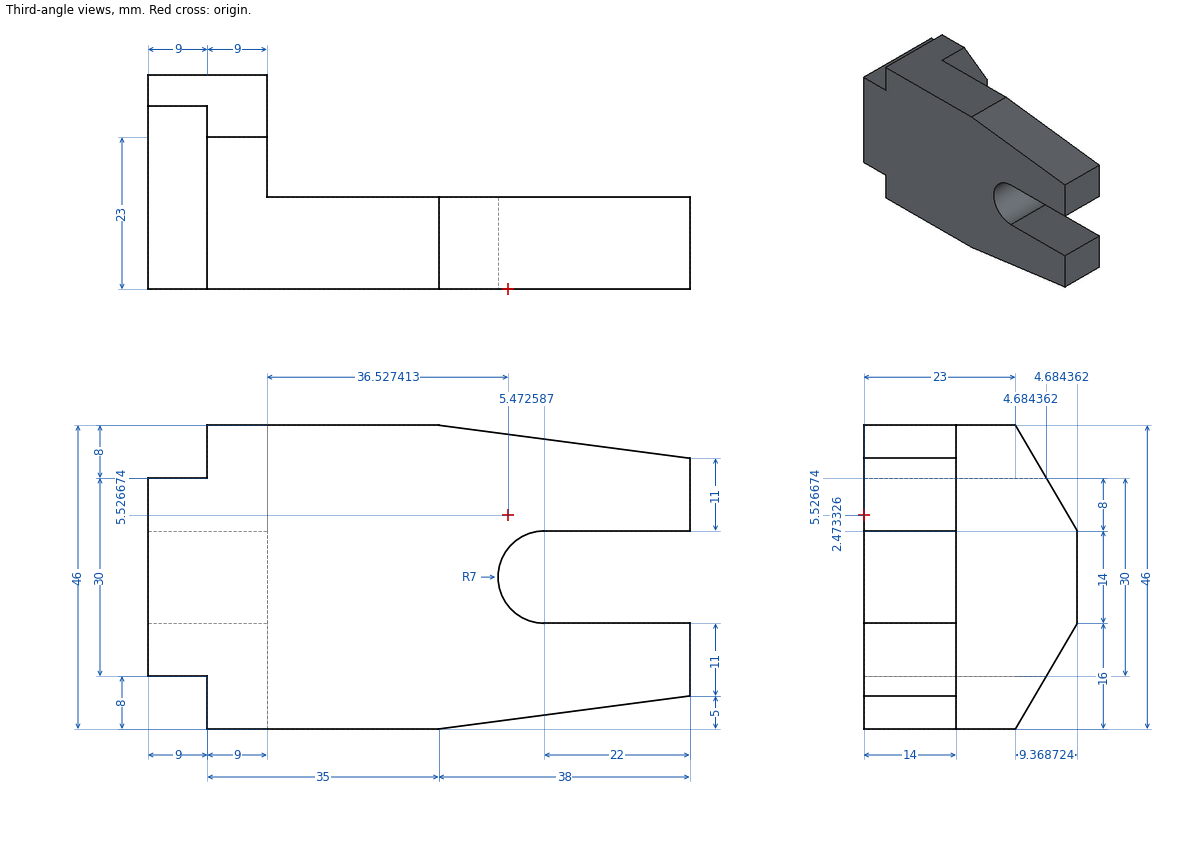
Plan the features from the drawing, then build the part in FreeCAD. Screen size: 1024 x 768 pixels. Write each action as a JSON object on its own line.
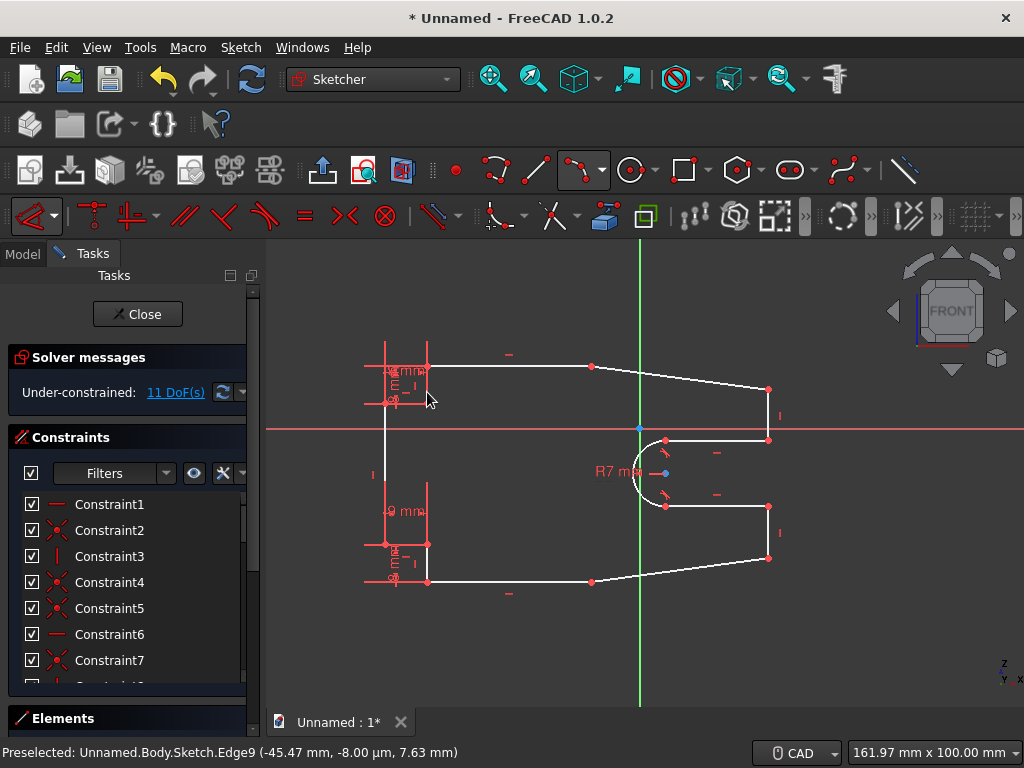
{"action": "left_click", "coordinate": [697, 506]}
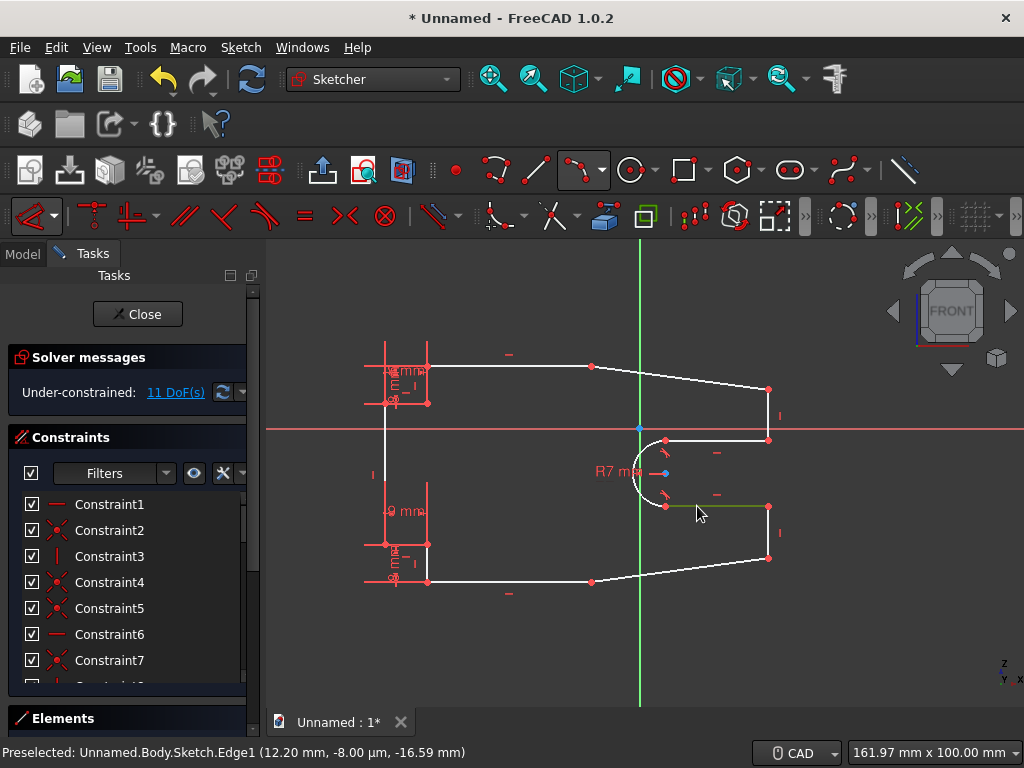
{"action": "key", "text": "l"}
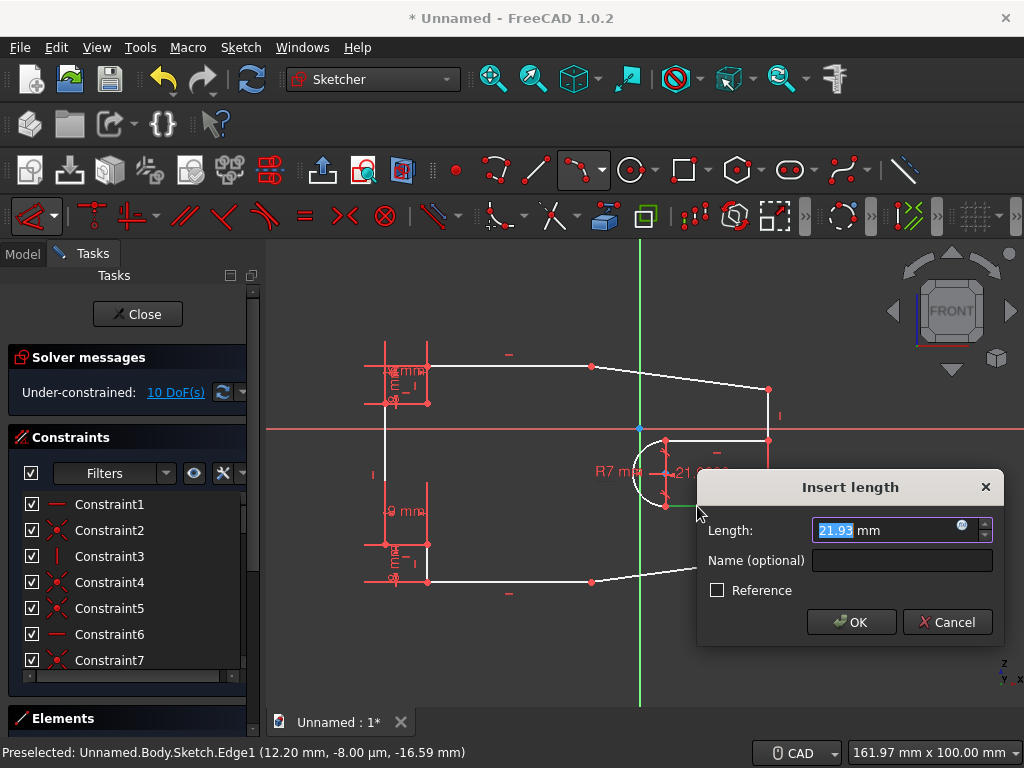
{"action": "type", "text": "22"}
{"action": "key", "text": "Return"}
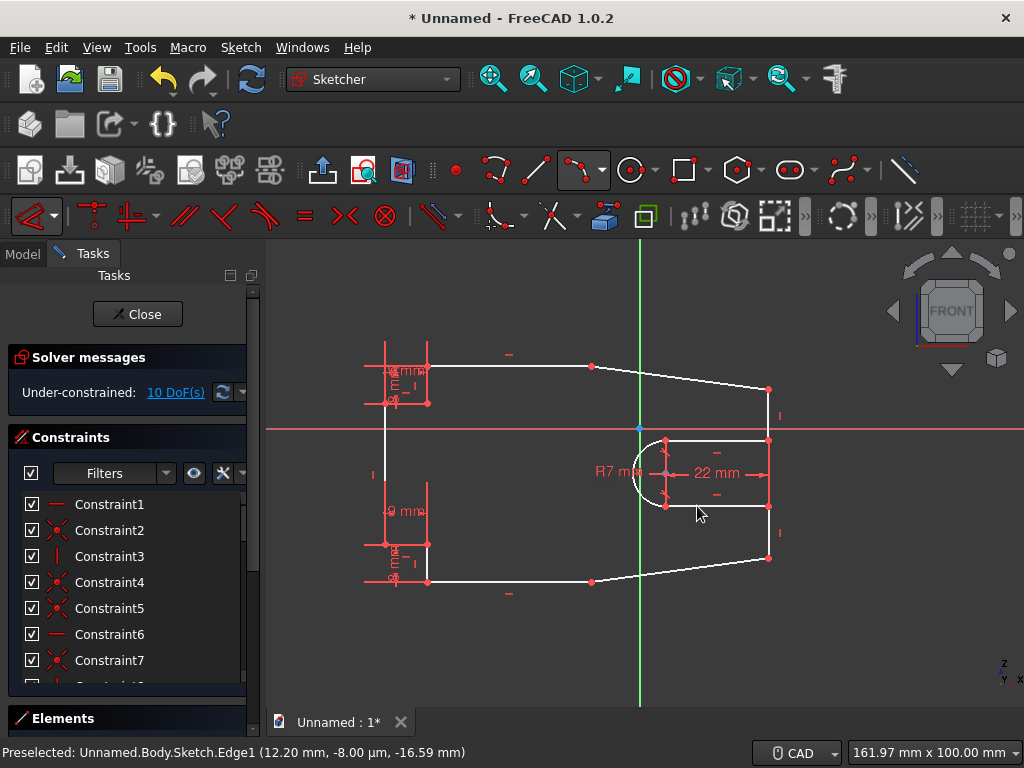
{"action": "left_click", "coordinate": [769, 522]}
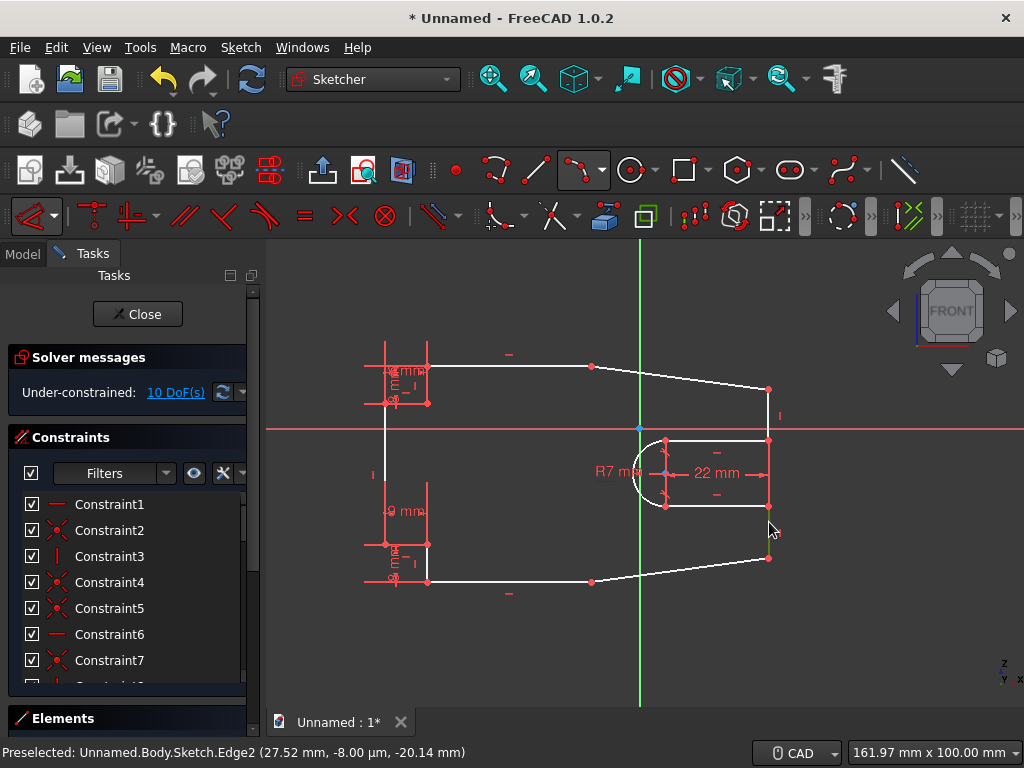
{"action": "left_click", "coordinate": [56, 216]}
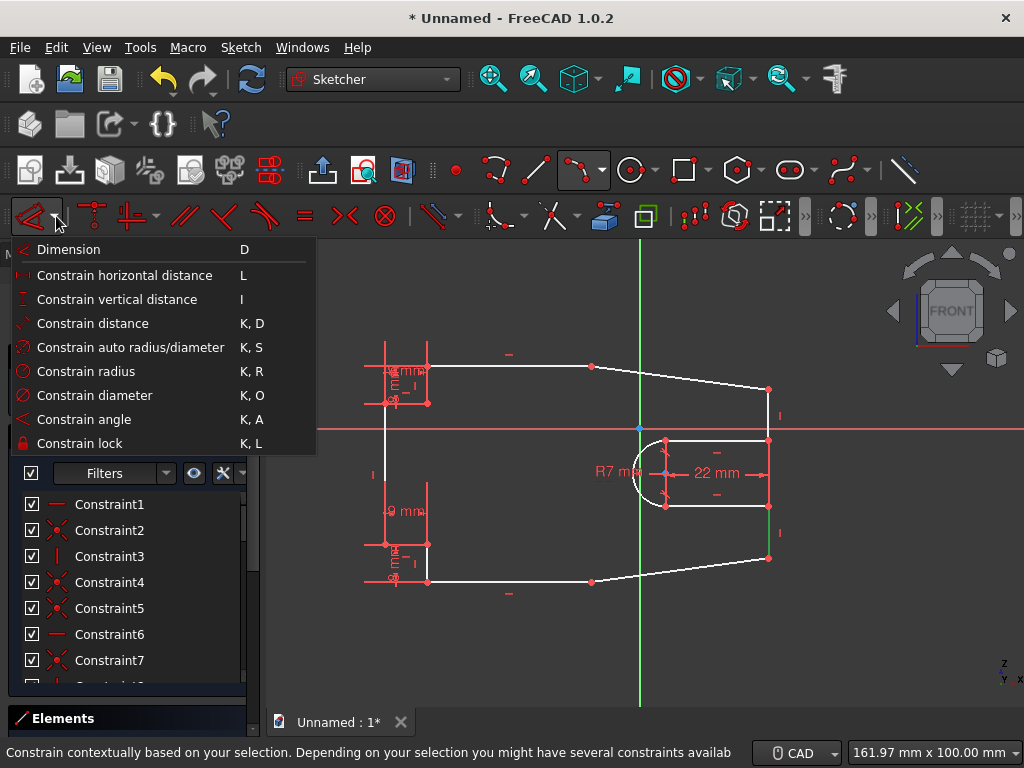
{"action": "left_click", "coordinate": [164, 299]}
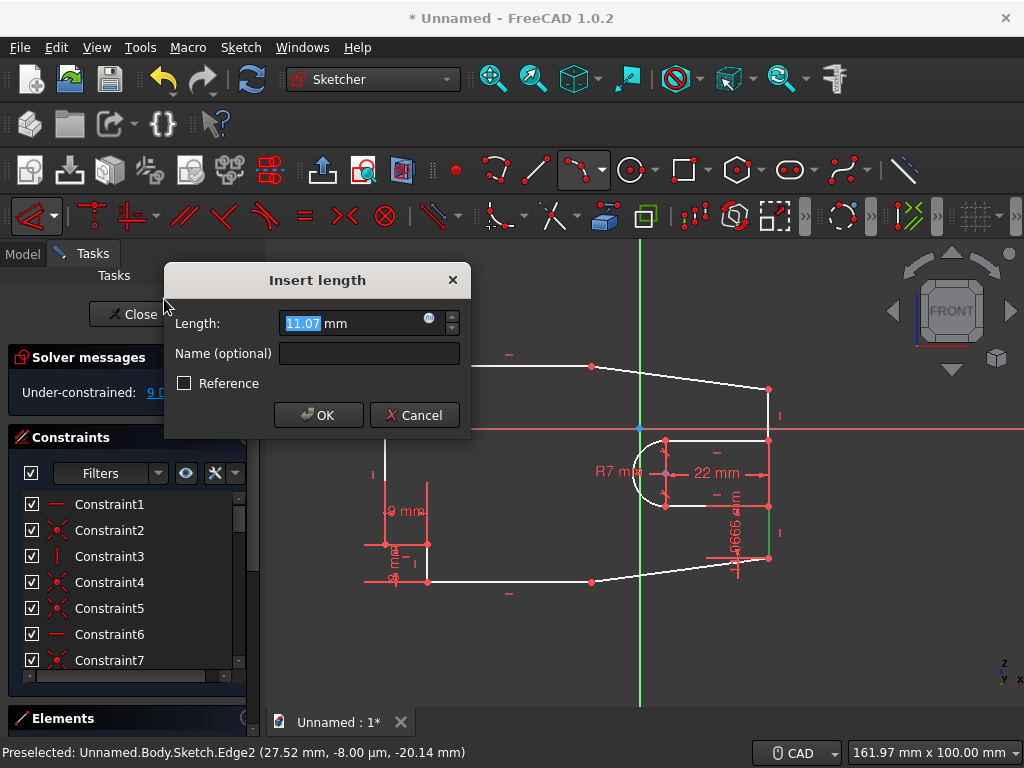
{"action": "type", "text": "11"}
{"action": "key", "text": "Return"}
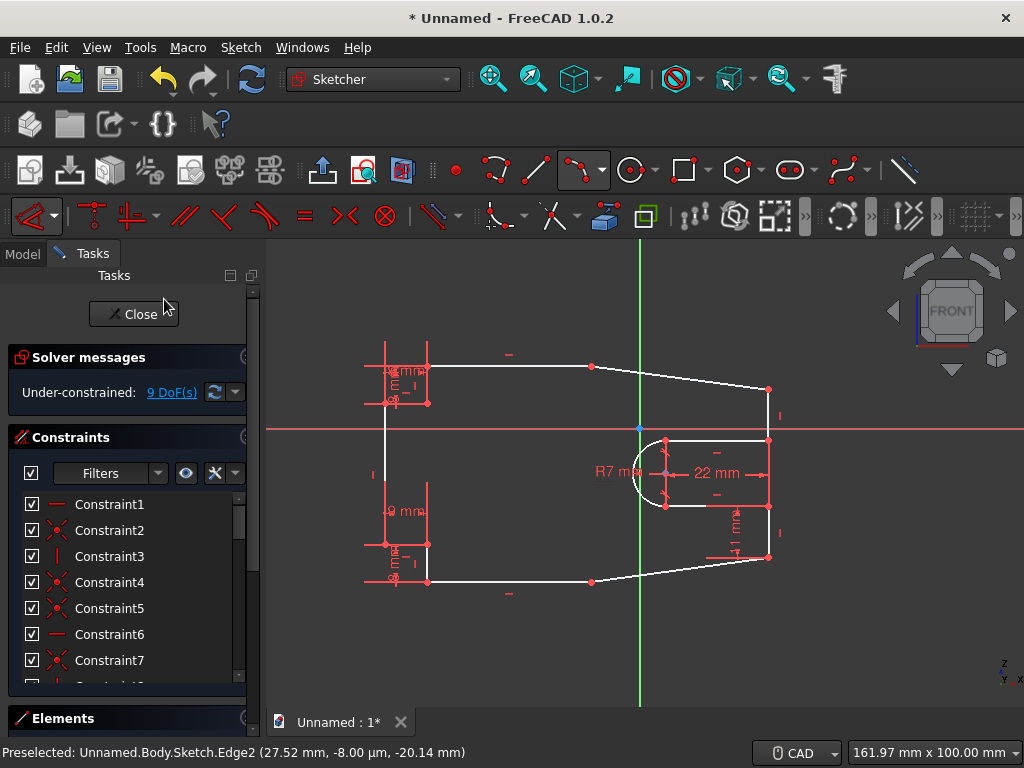
{"action": "left_click", "coordinate": [542, 582]}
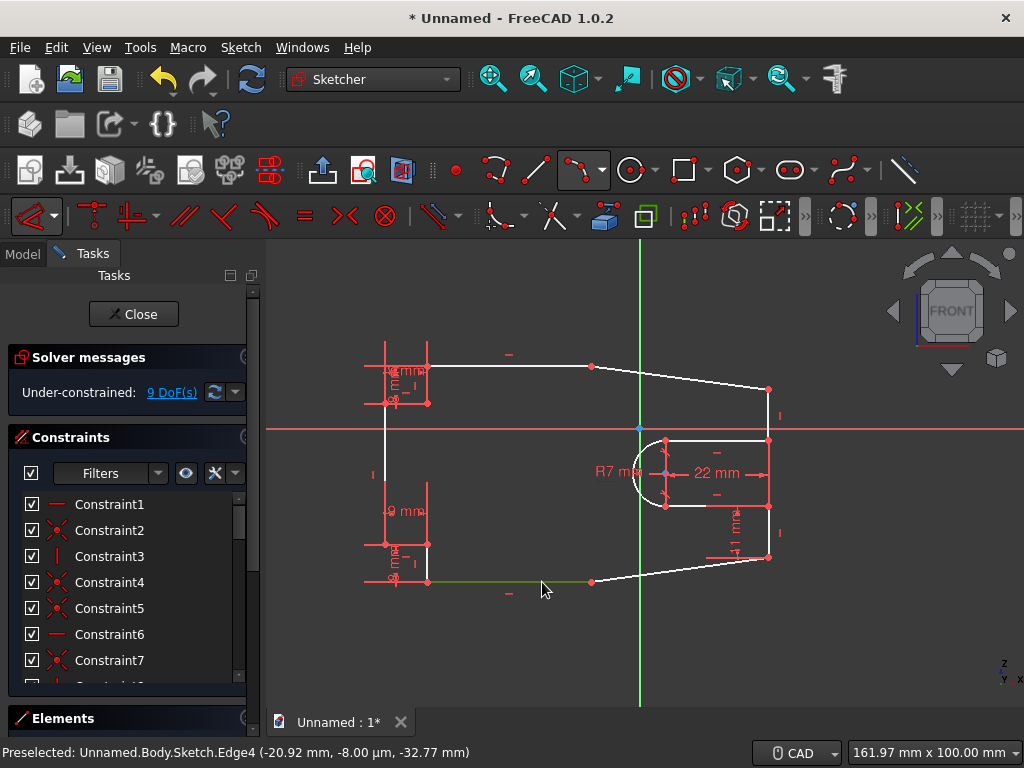
{"action": "left_click", "coordinate": [56, 216]}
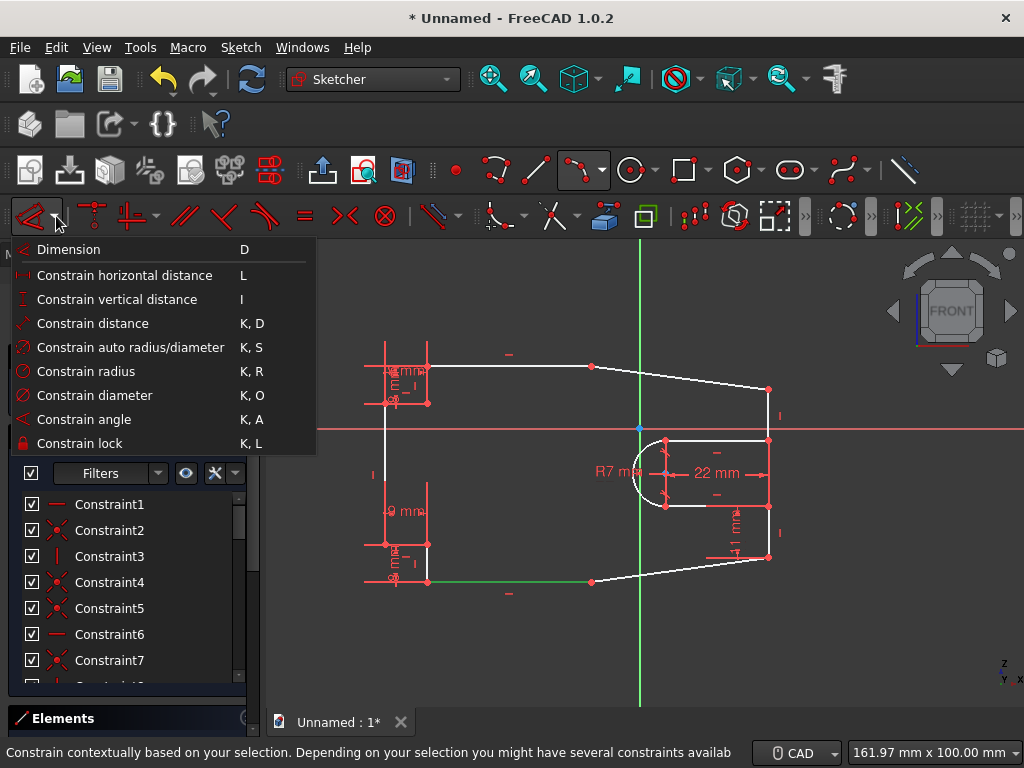
{"action": "left_click", "coordinate": [164, 275]}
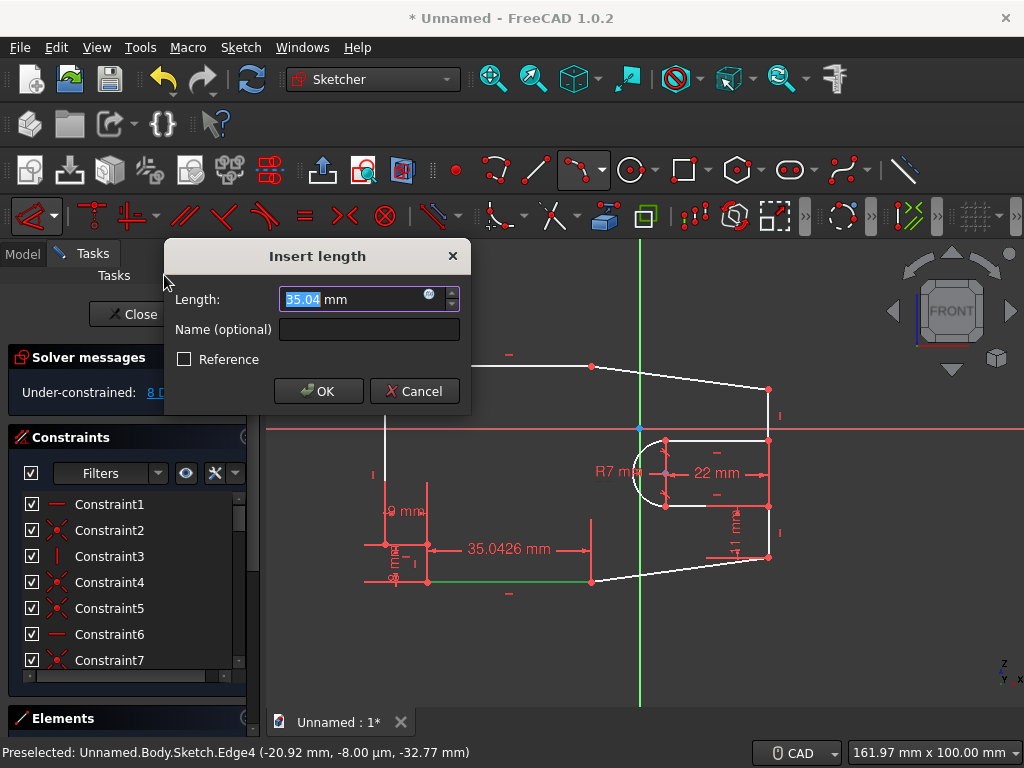
{"action": "type", "text": "35"}
{"action": "key", "text": "Return"}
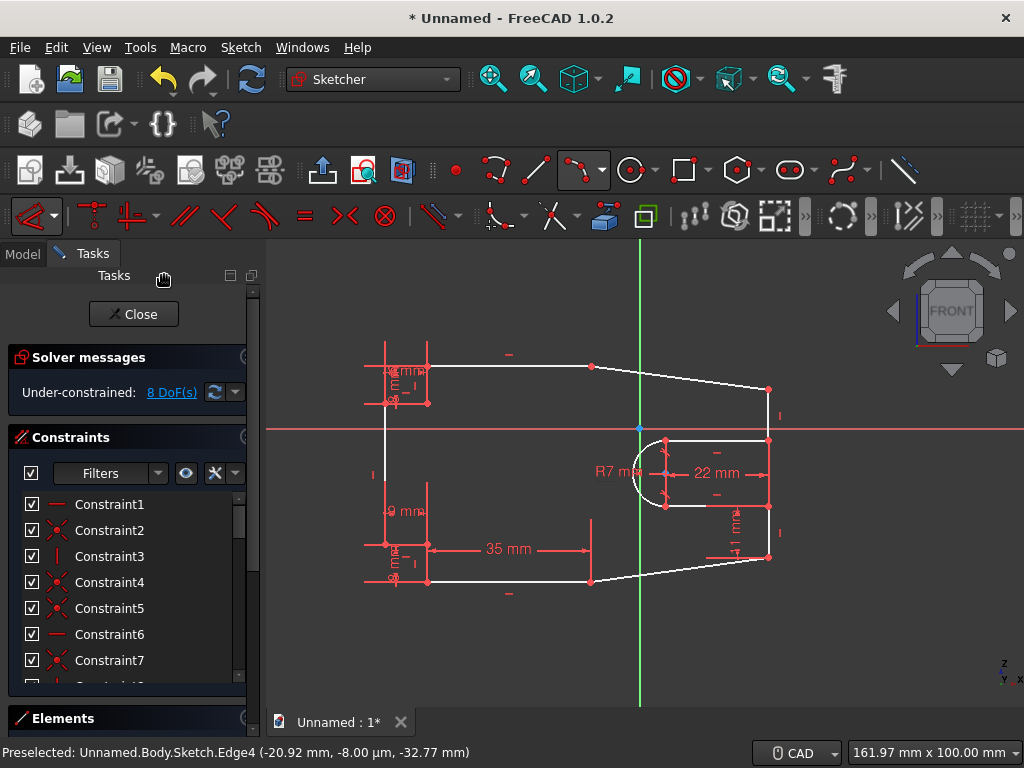
{"action": "left_click", "coordinate": [385, 502]}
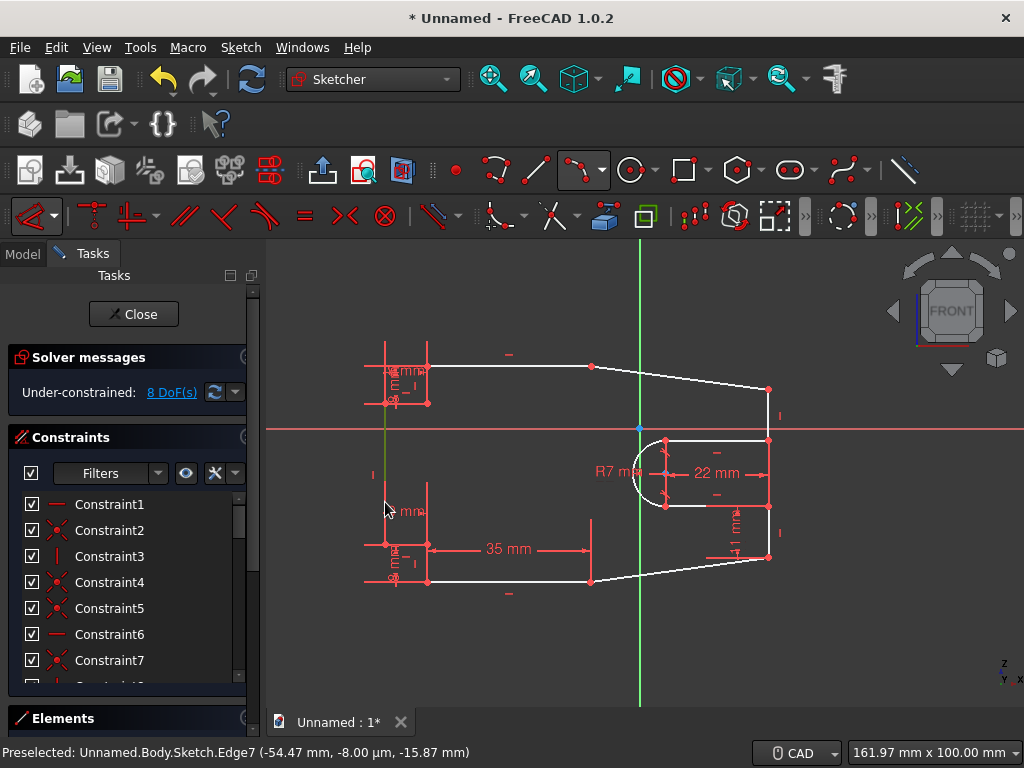
{"action": "left_click", "coordinate": [56, 216]}